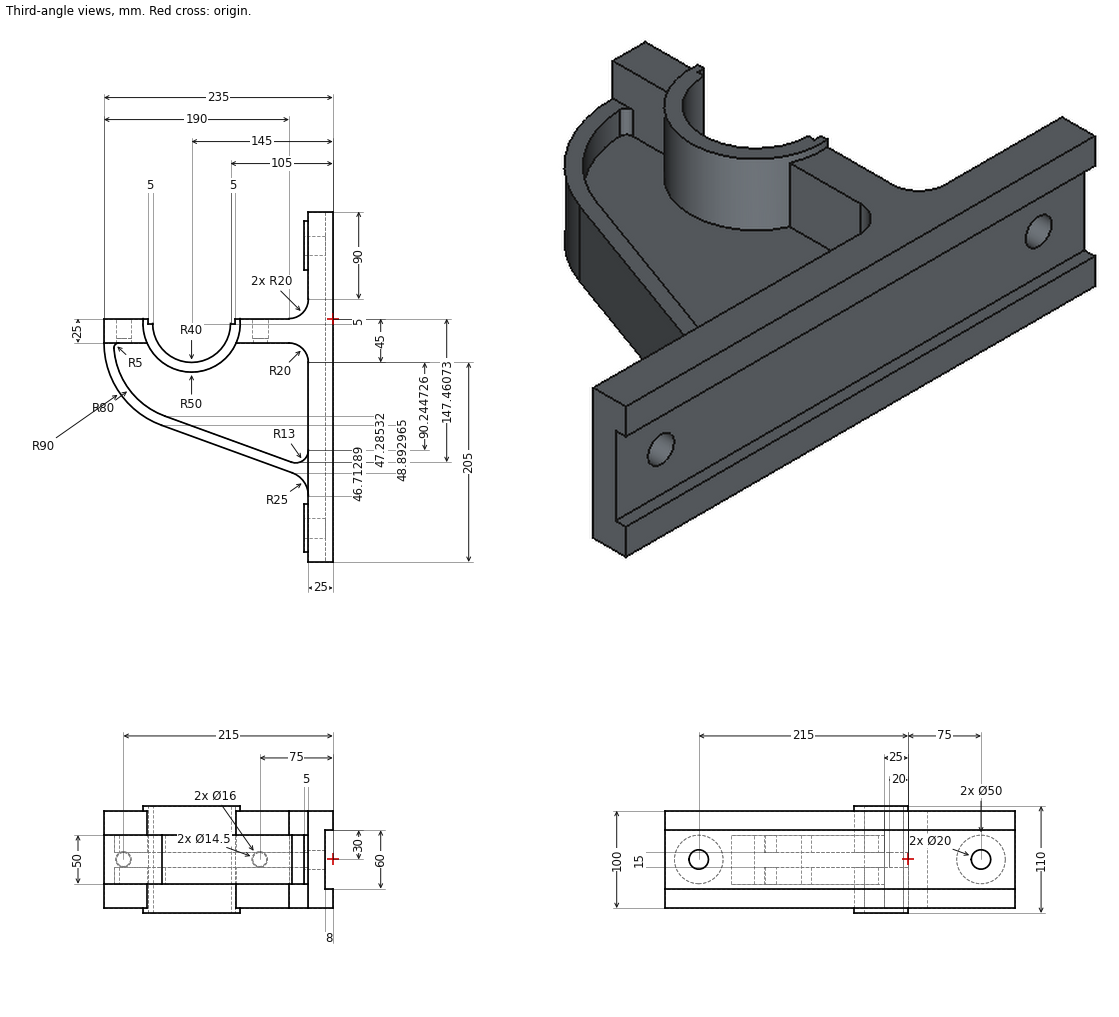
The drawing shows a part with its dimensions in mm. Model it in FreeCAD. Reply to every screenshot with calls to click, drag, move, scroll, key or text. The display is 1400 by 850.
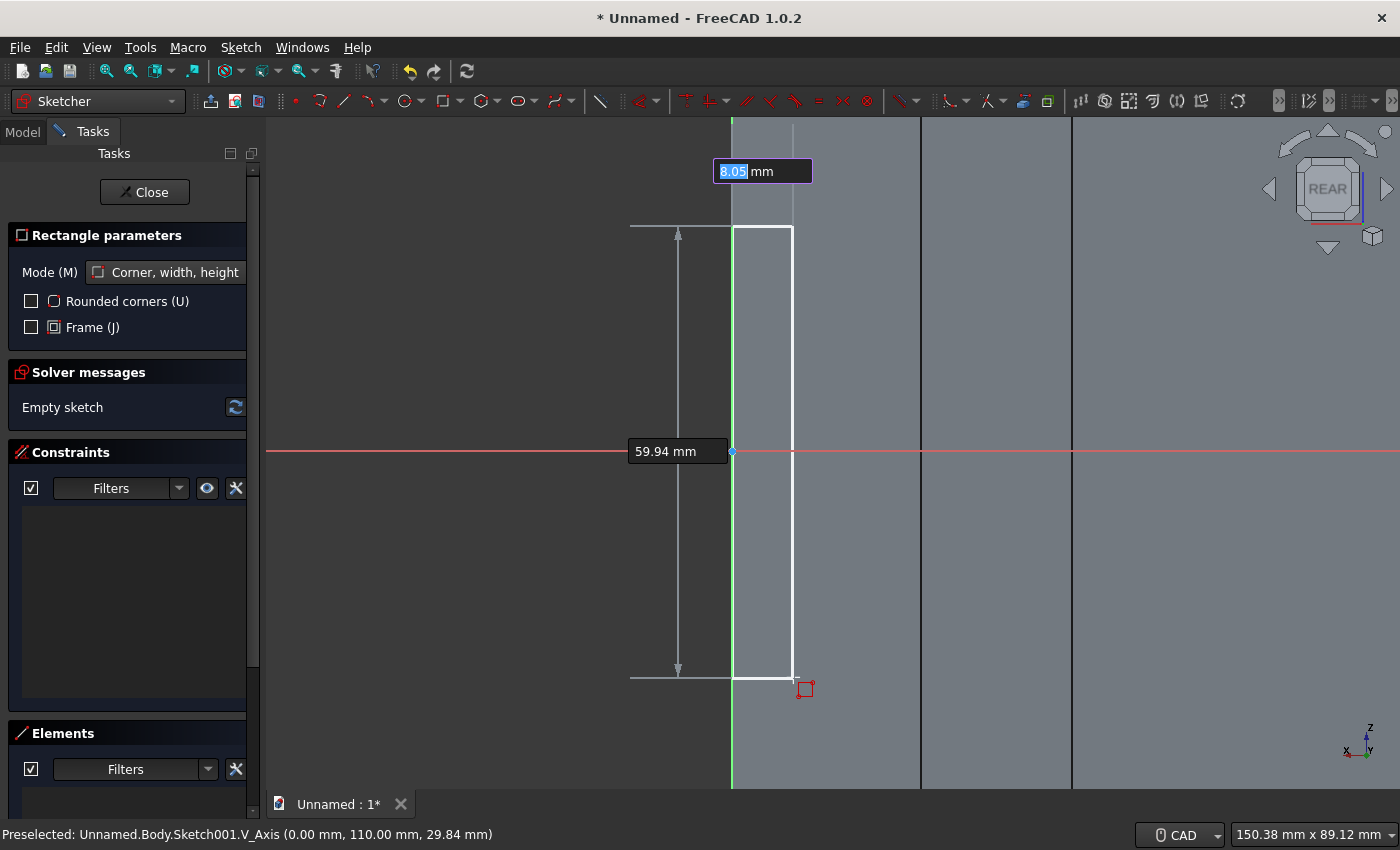
text(8)
key(Tab)
text(60)
key(Return)
key(Escape)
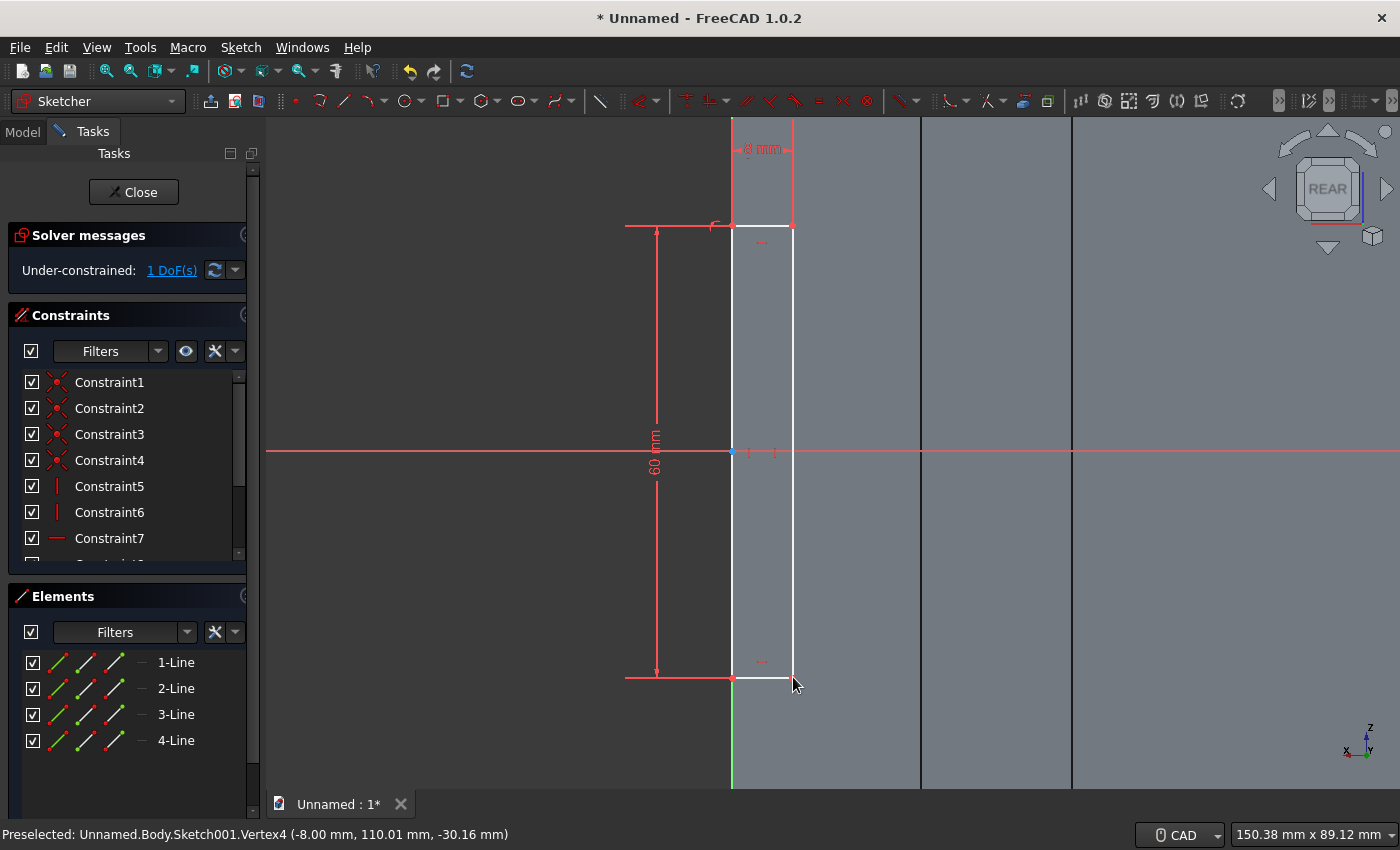
click(640, 102)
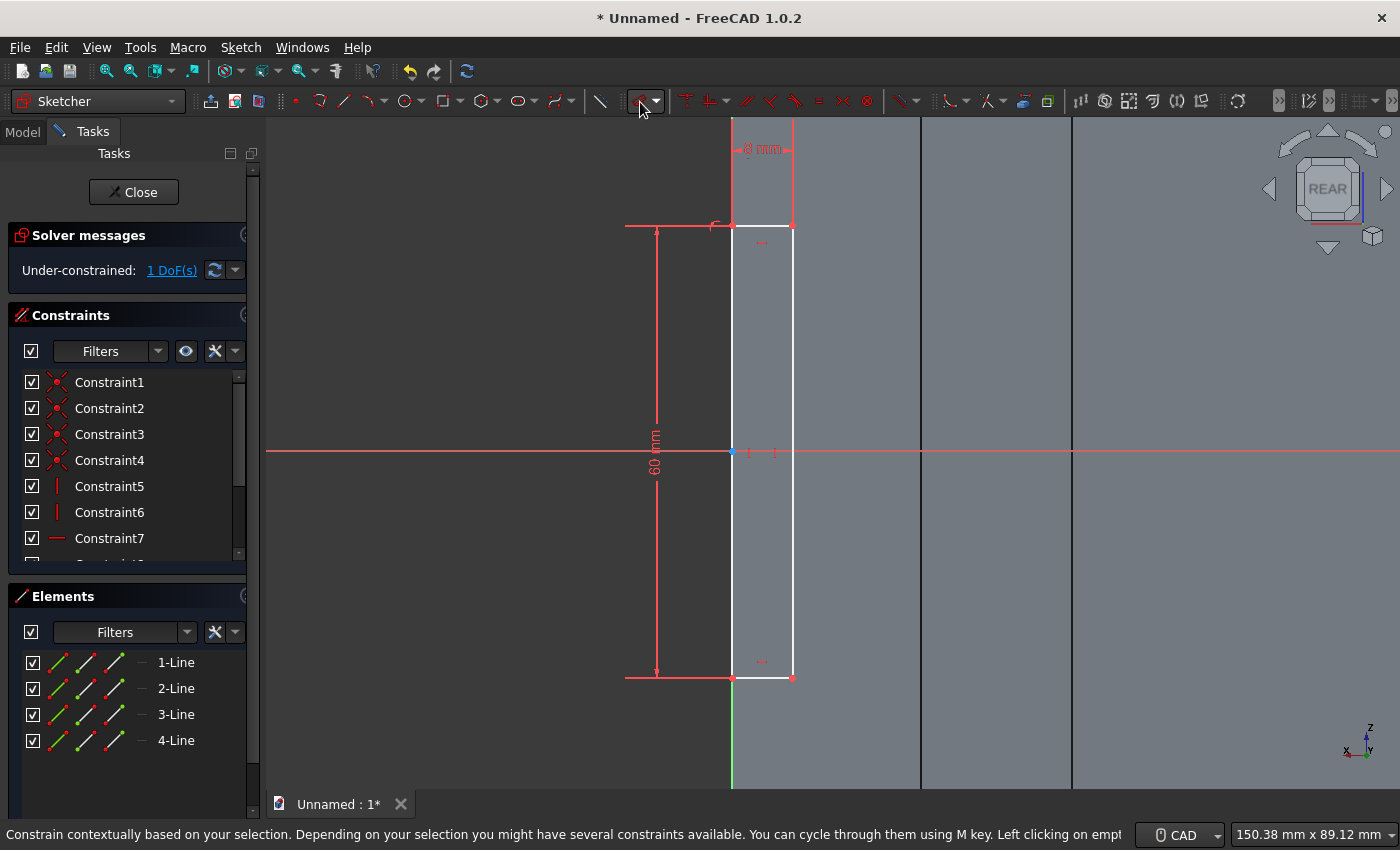
click(732, 226)
click(698, 339)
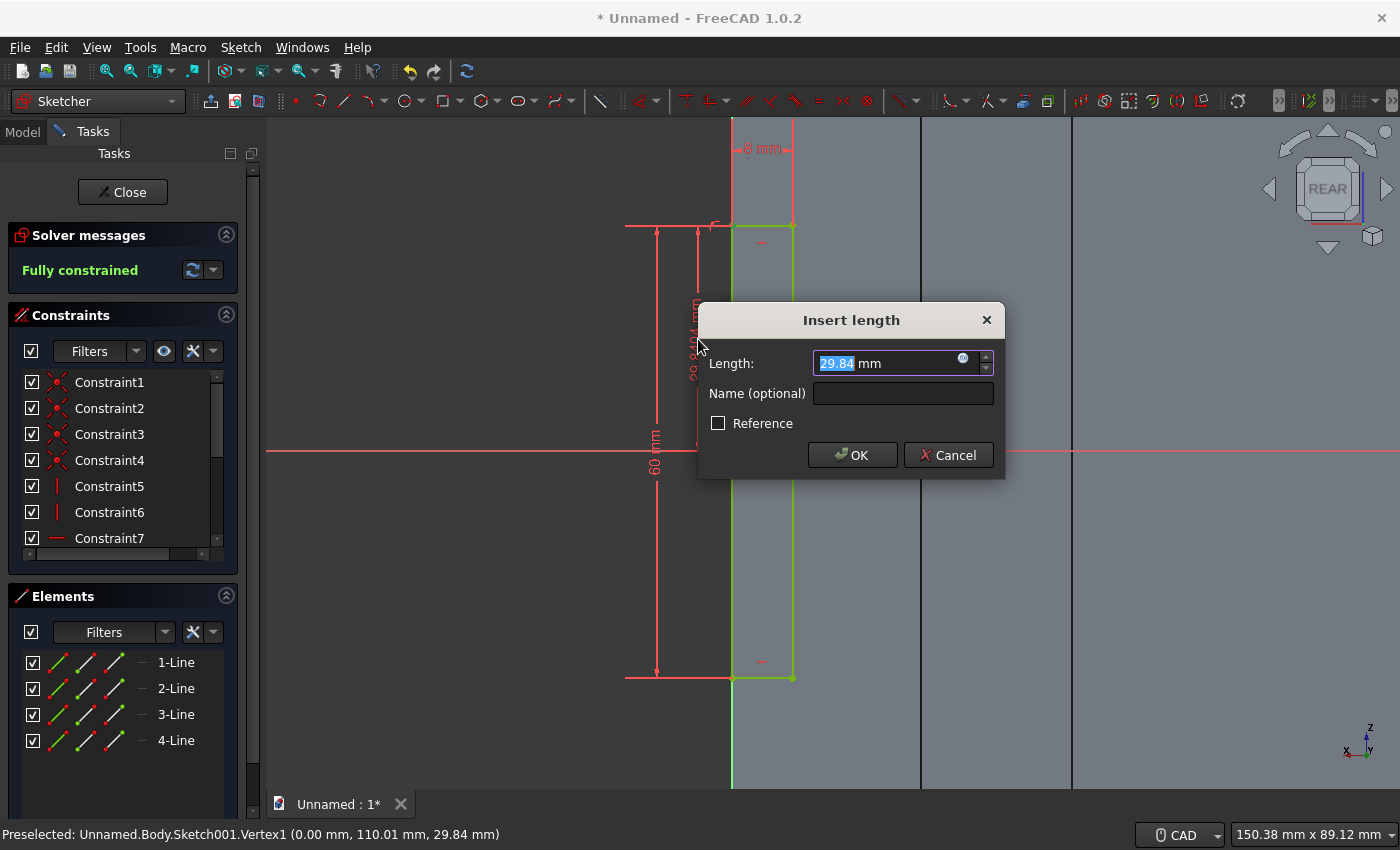
text(30)
key(Return)
key(Escape)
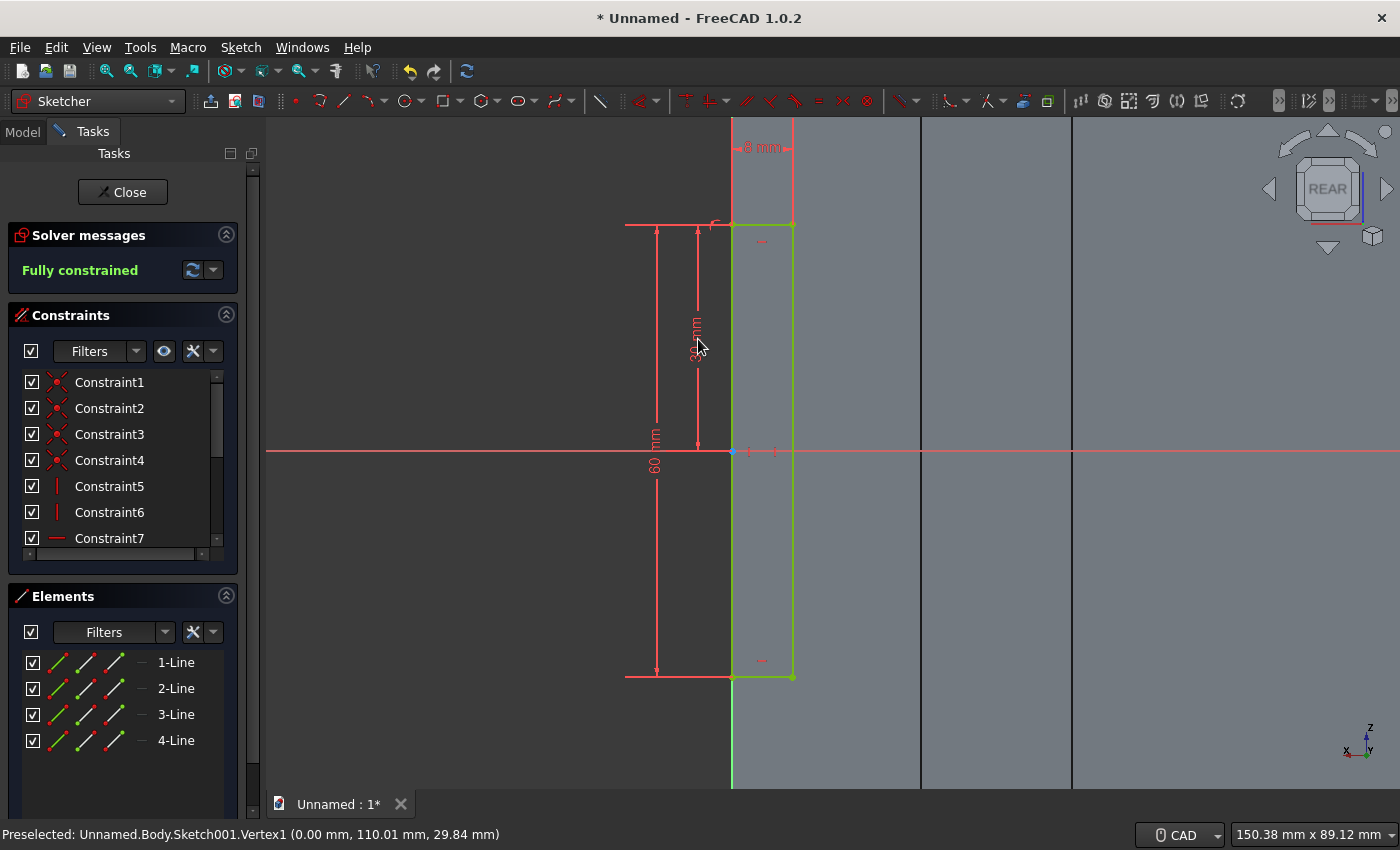
click(123, 192)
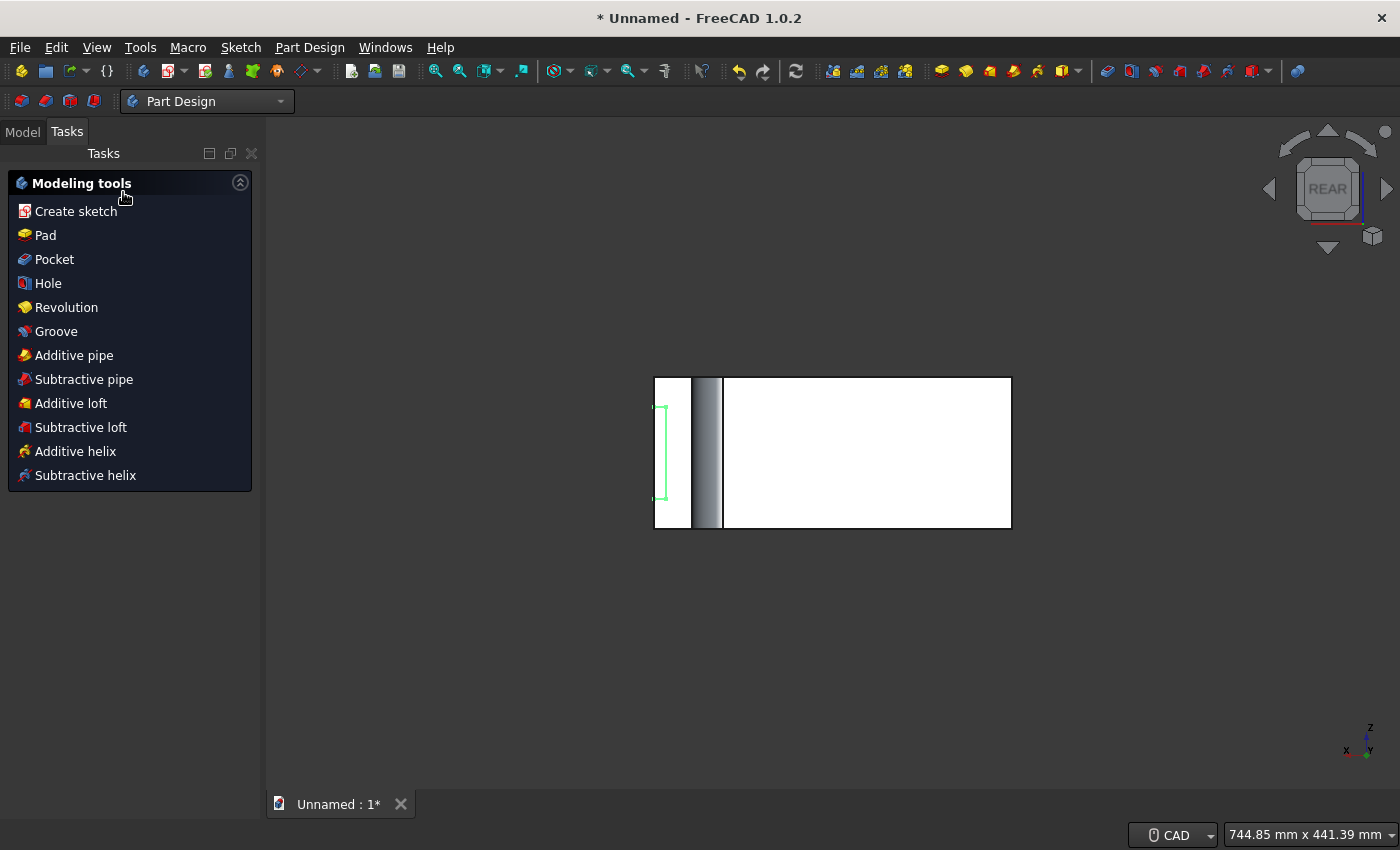
click(1108, 72)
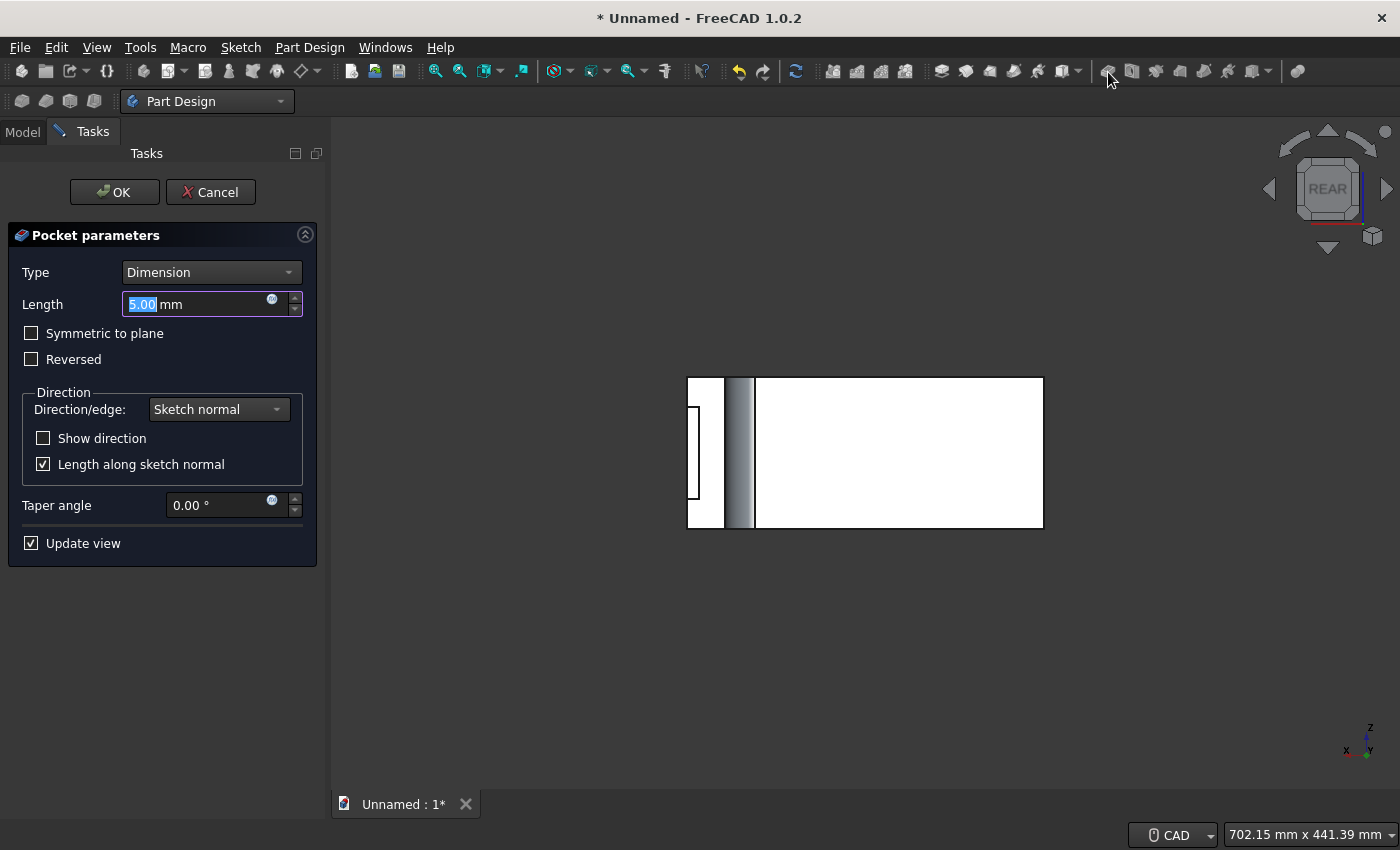
click(212, 272)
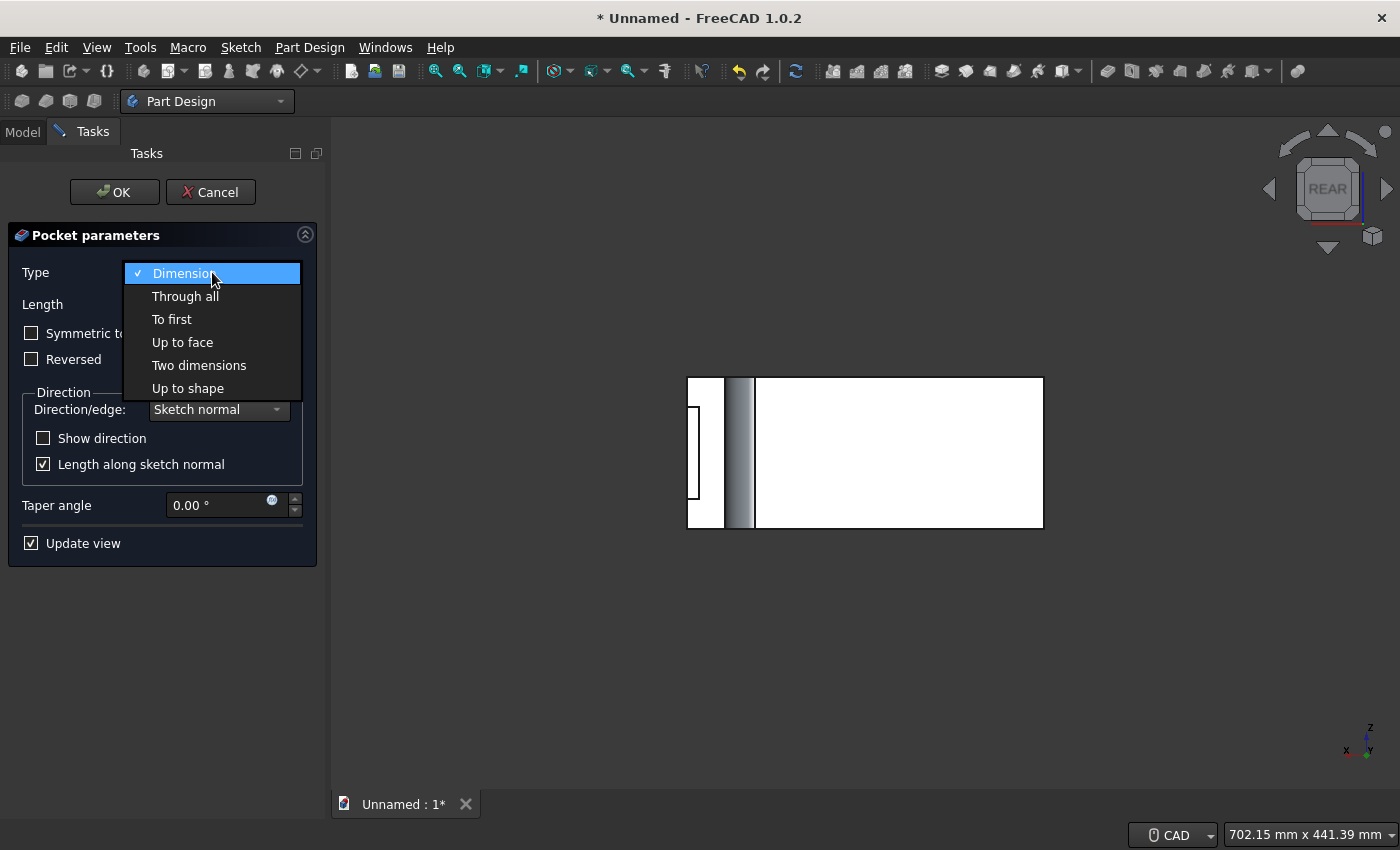
click(212, 296)